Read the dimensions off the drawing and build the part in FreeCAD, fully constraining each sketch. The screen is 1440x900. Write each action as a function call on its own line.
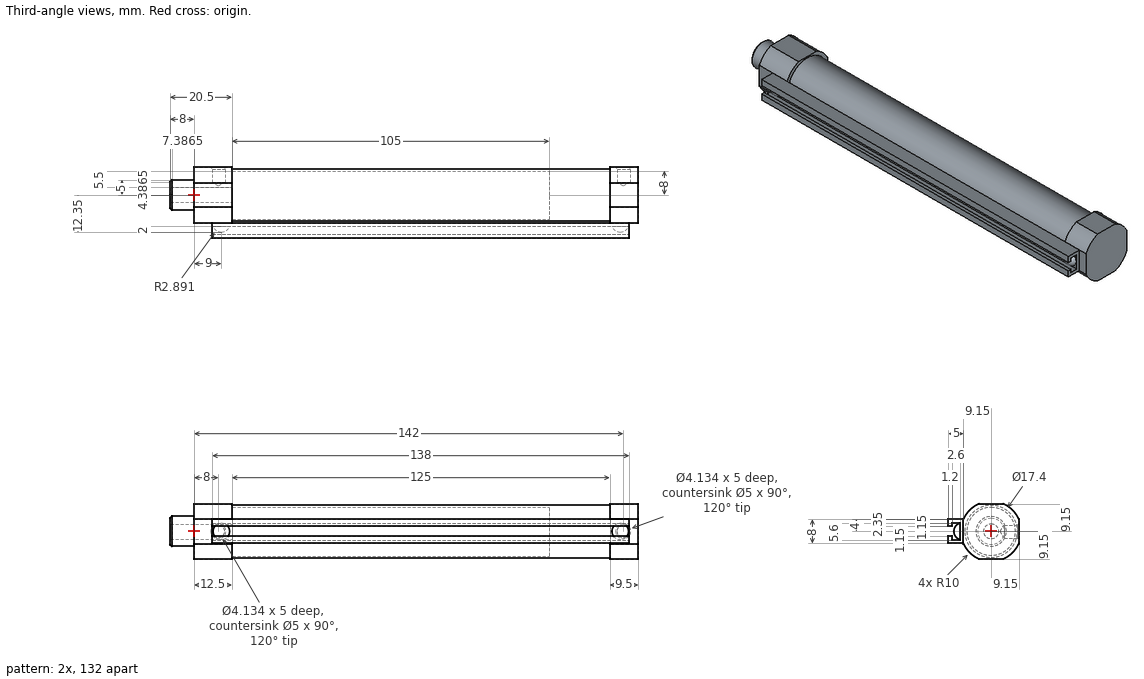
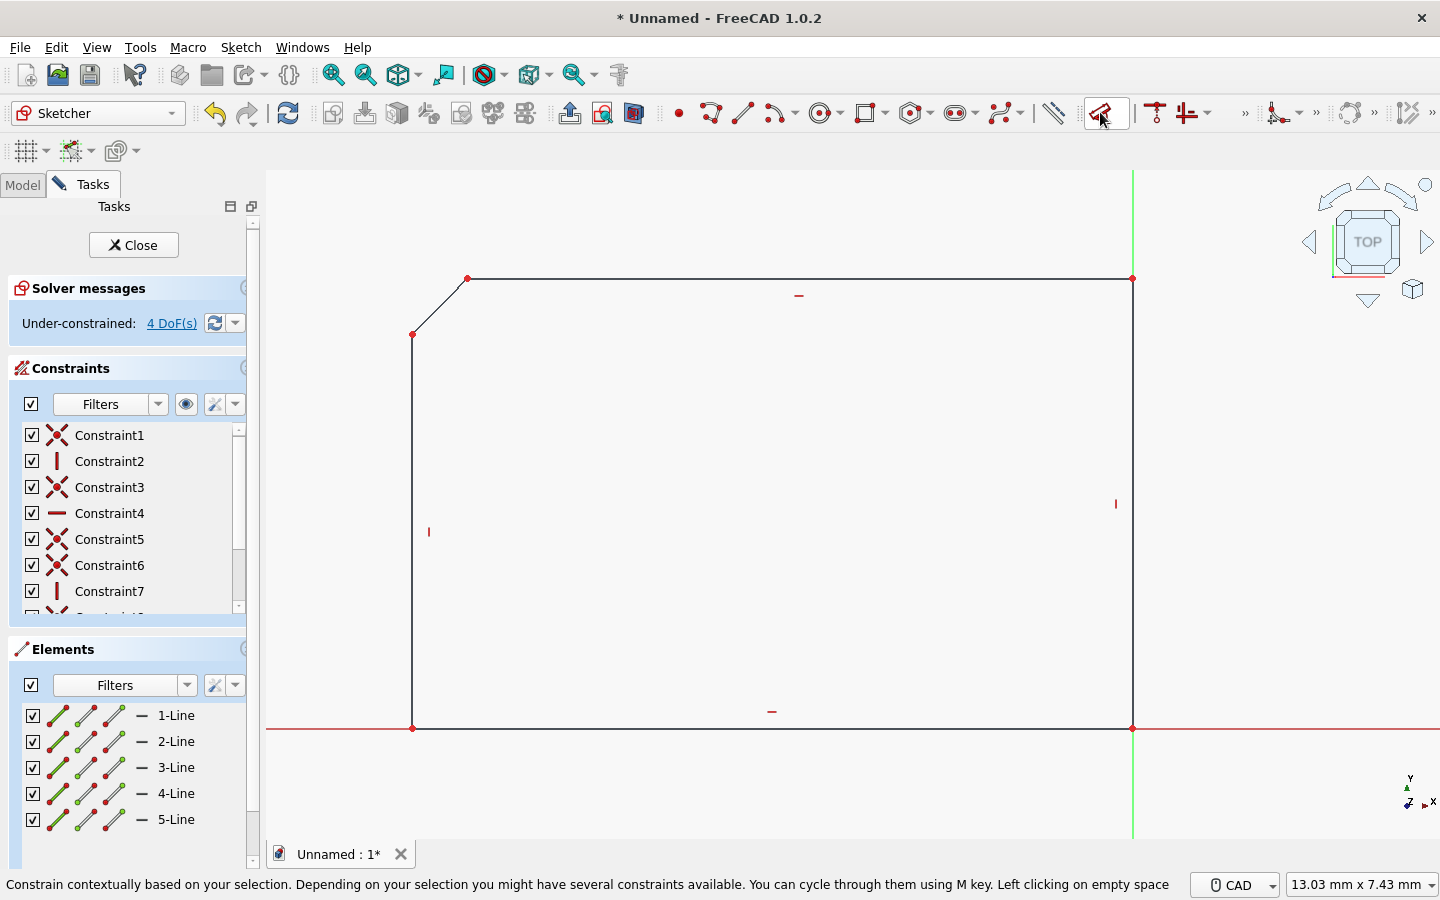
click(1133, 594)
click(1167, 504)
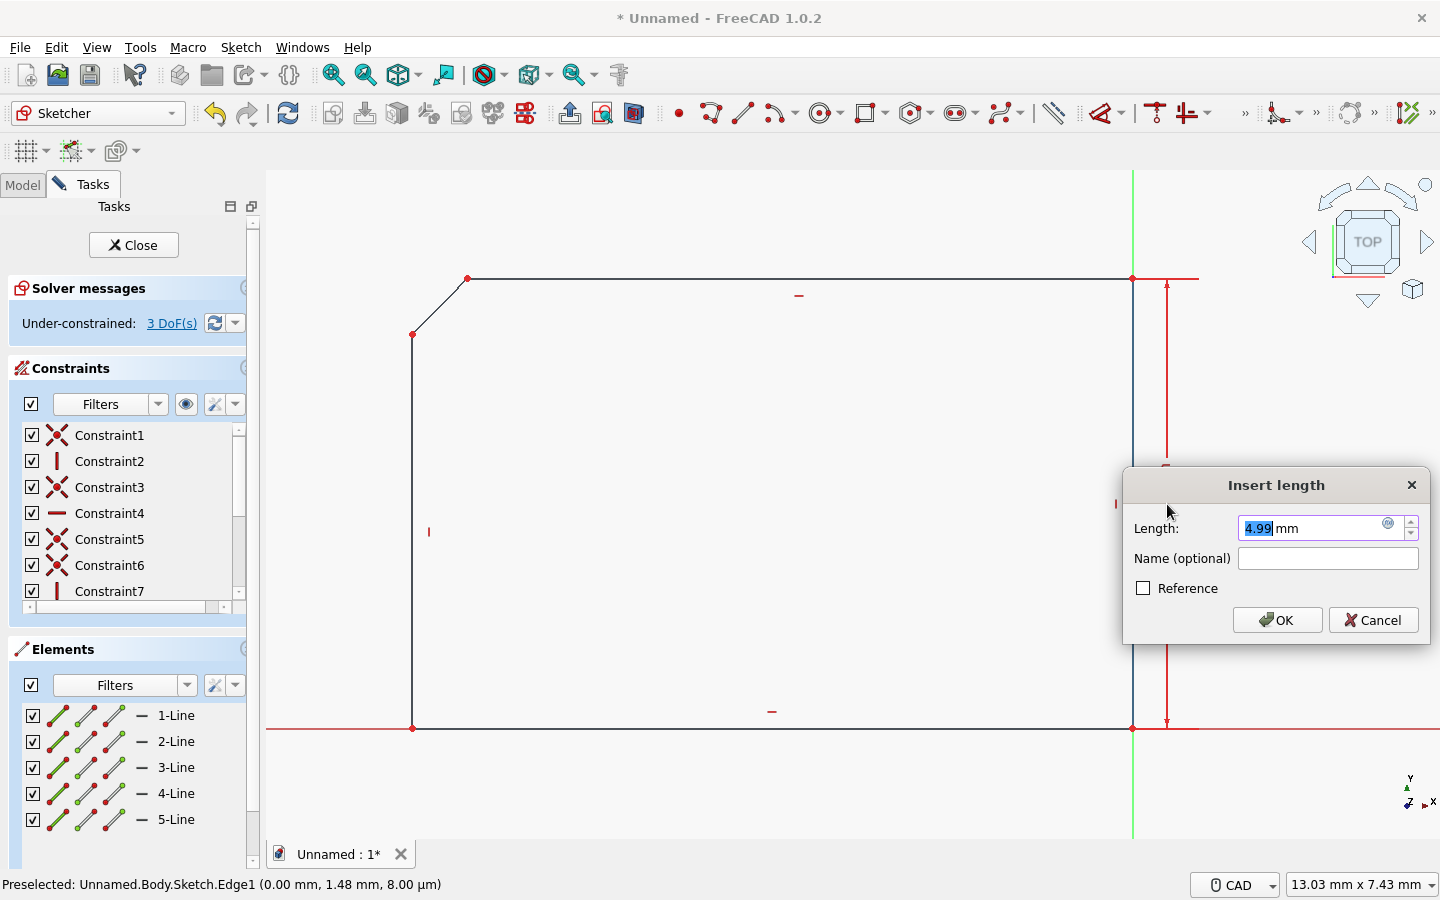
text(5)
key(Return)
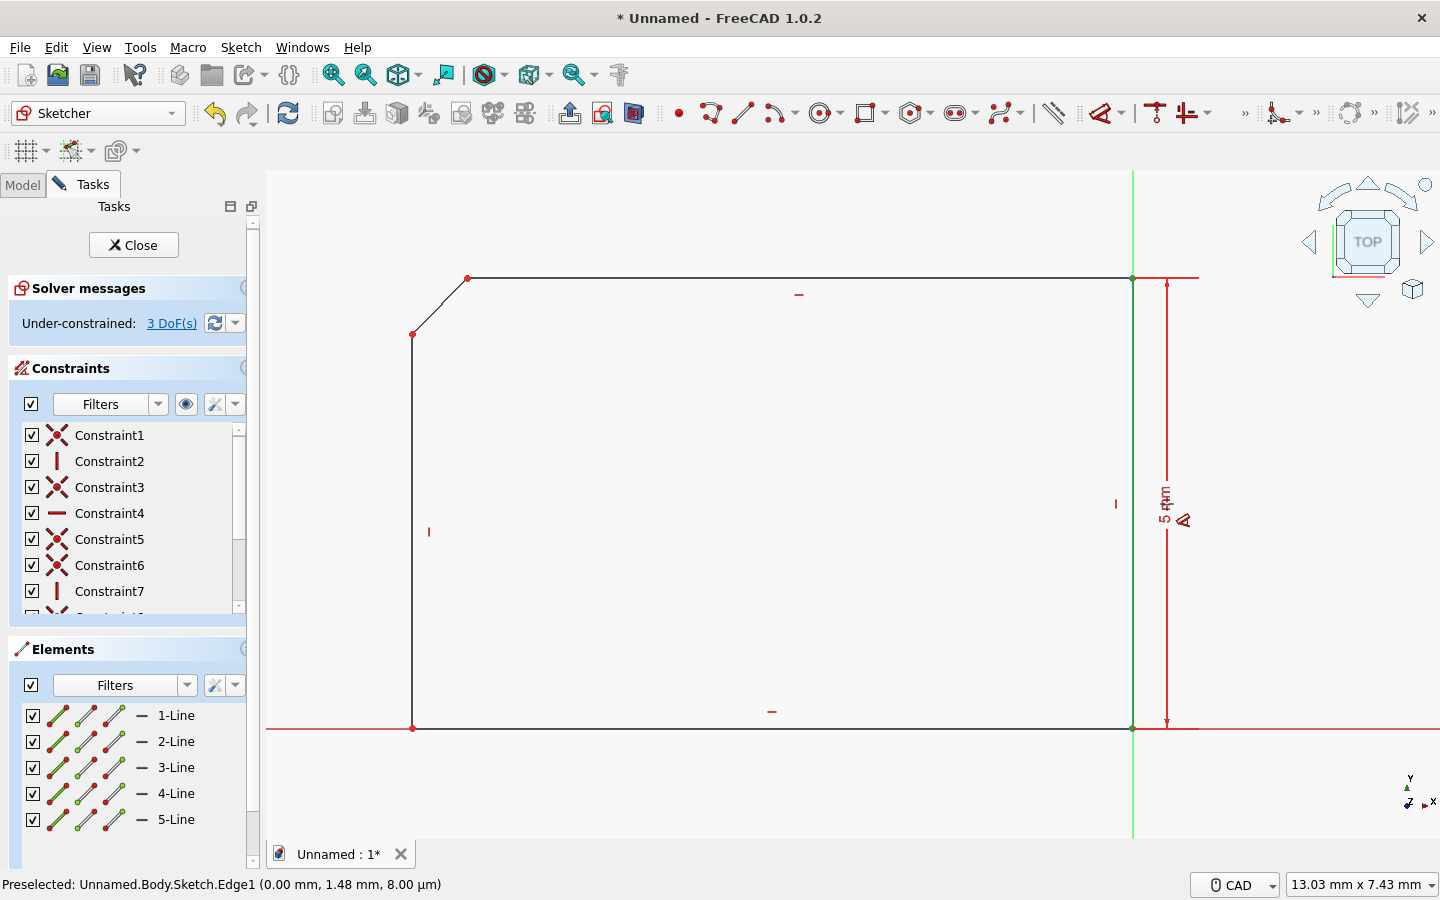
click(628, 729)
click(773, 763)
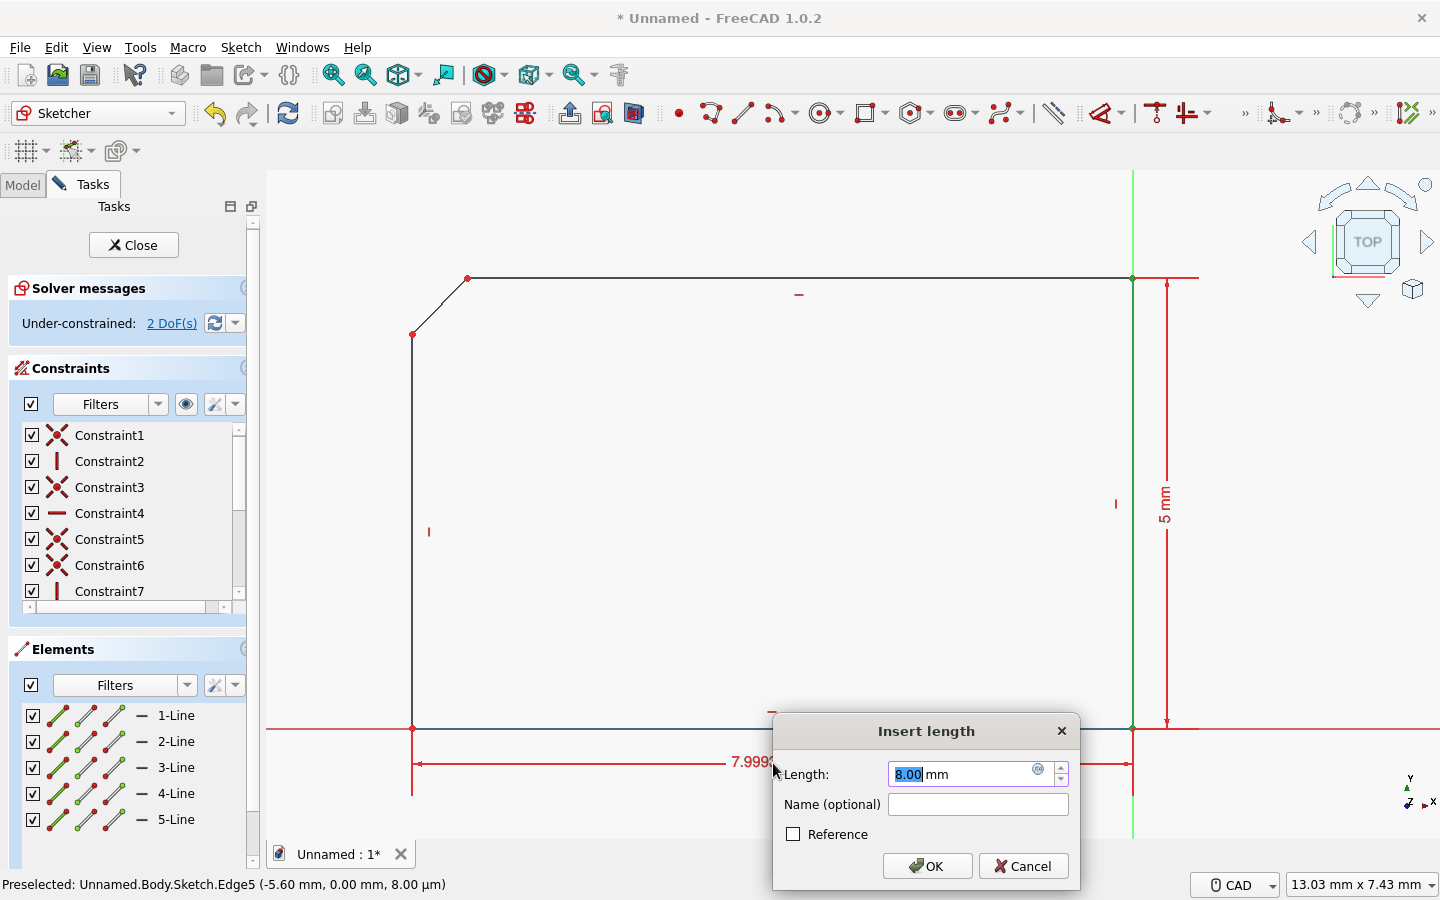
text(8)
key(Return)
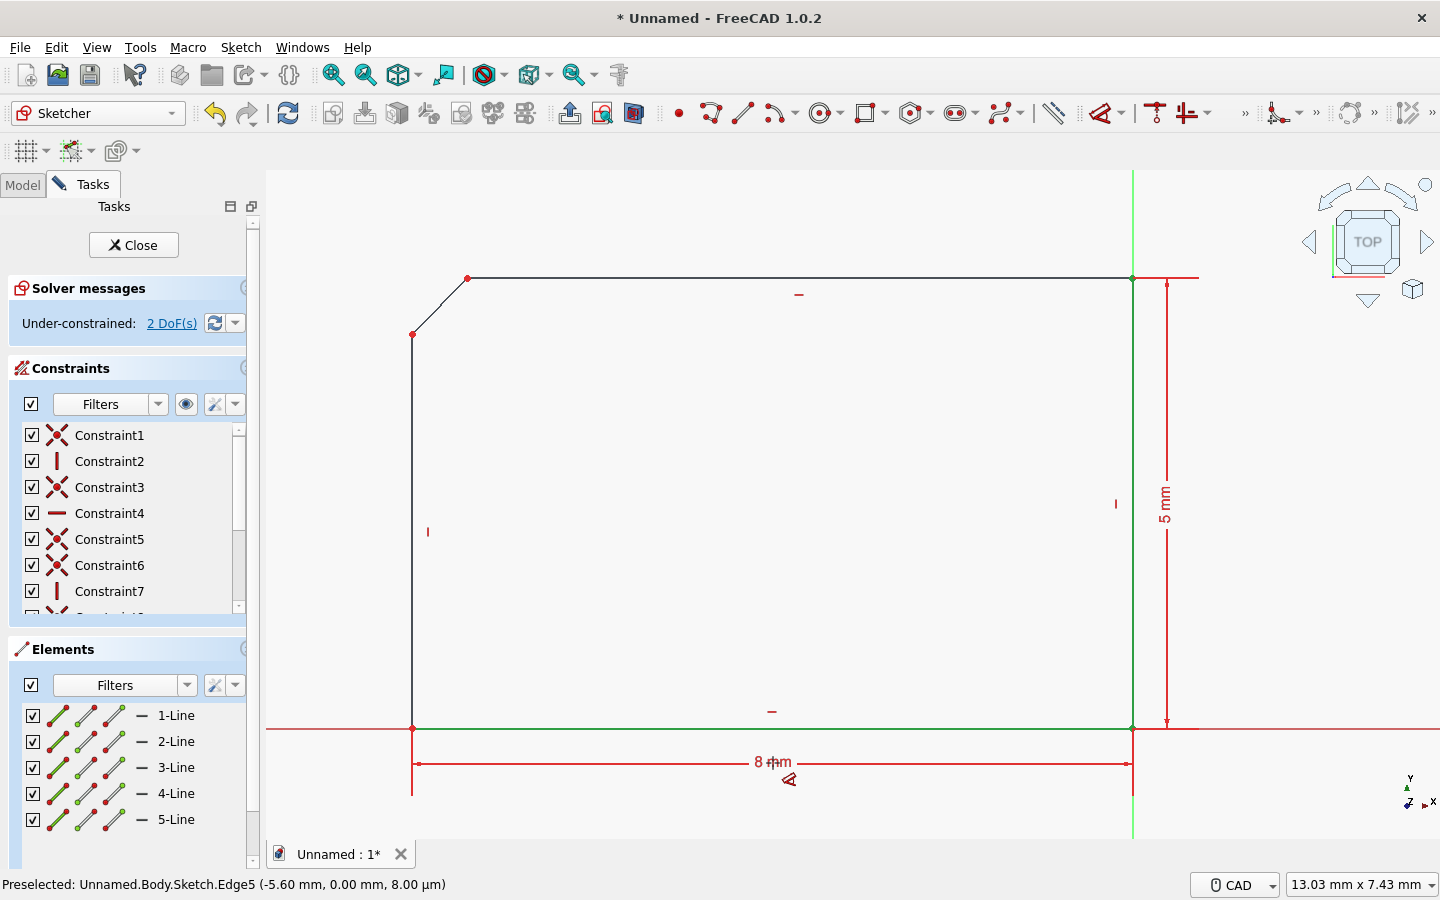
click(933, 278)
click(800, 244)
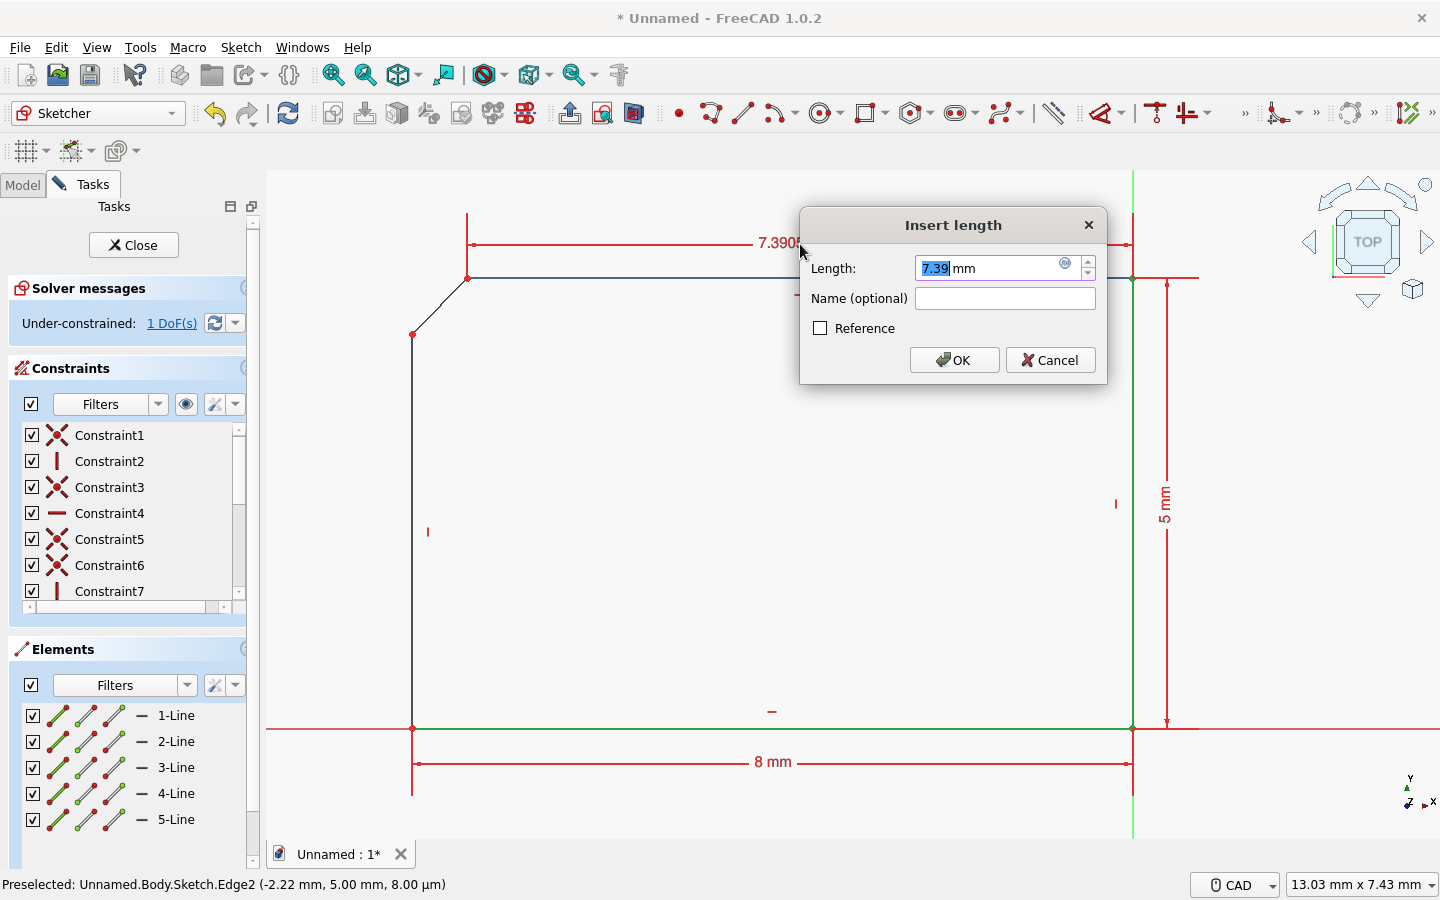
text(7.3865)
key(Return)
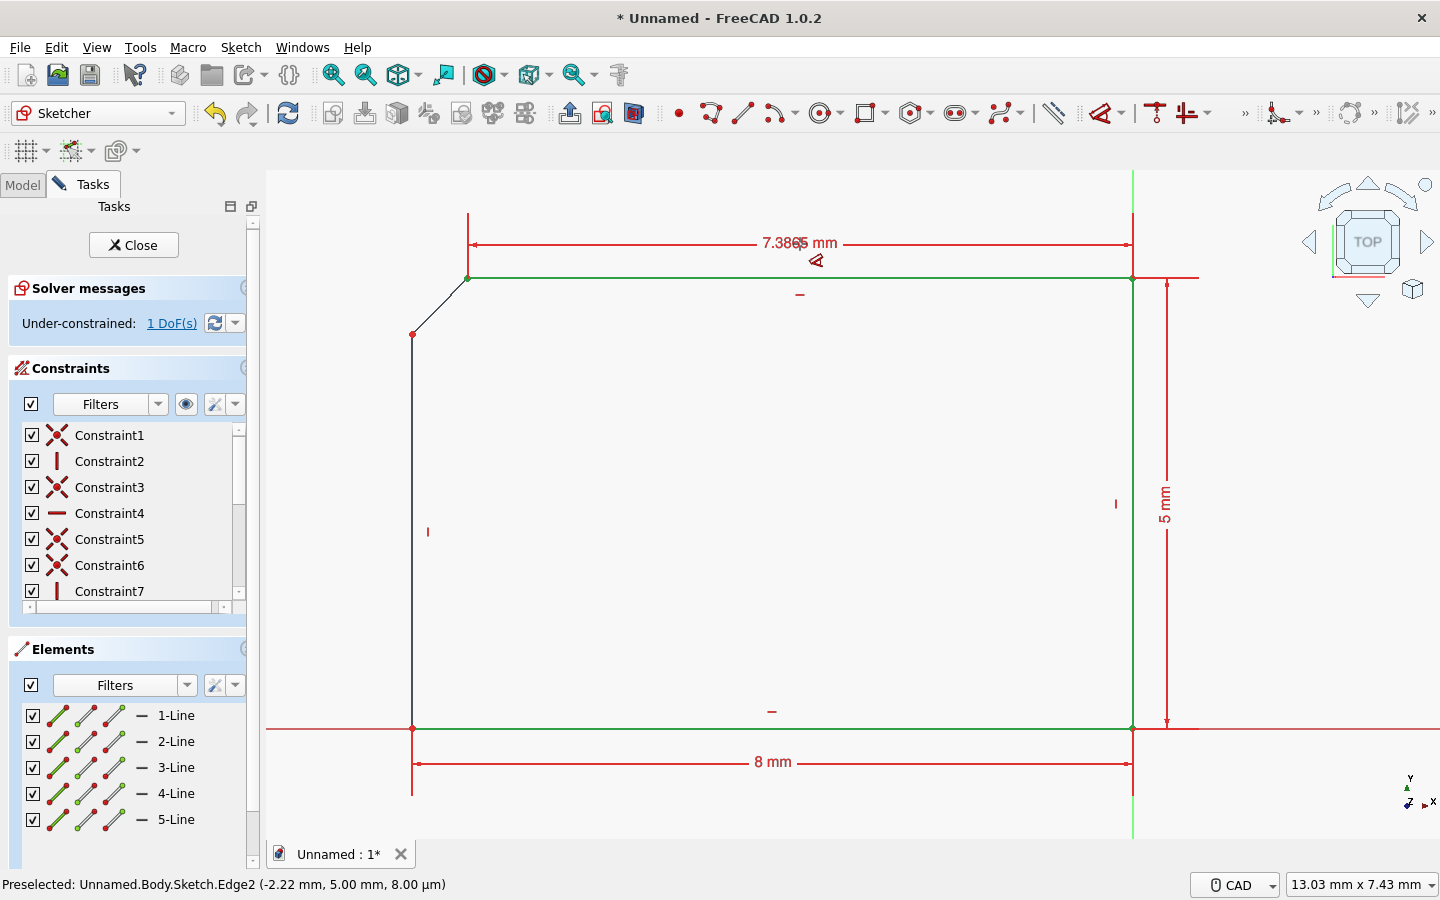
click(412, 453)
click(378, 532)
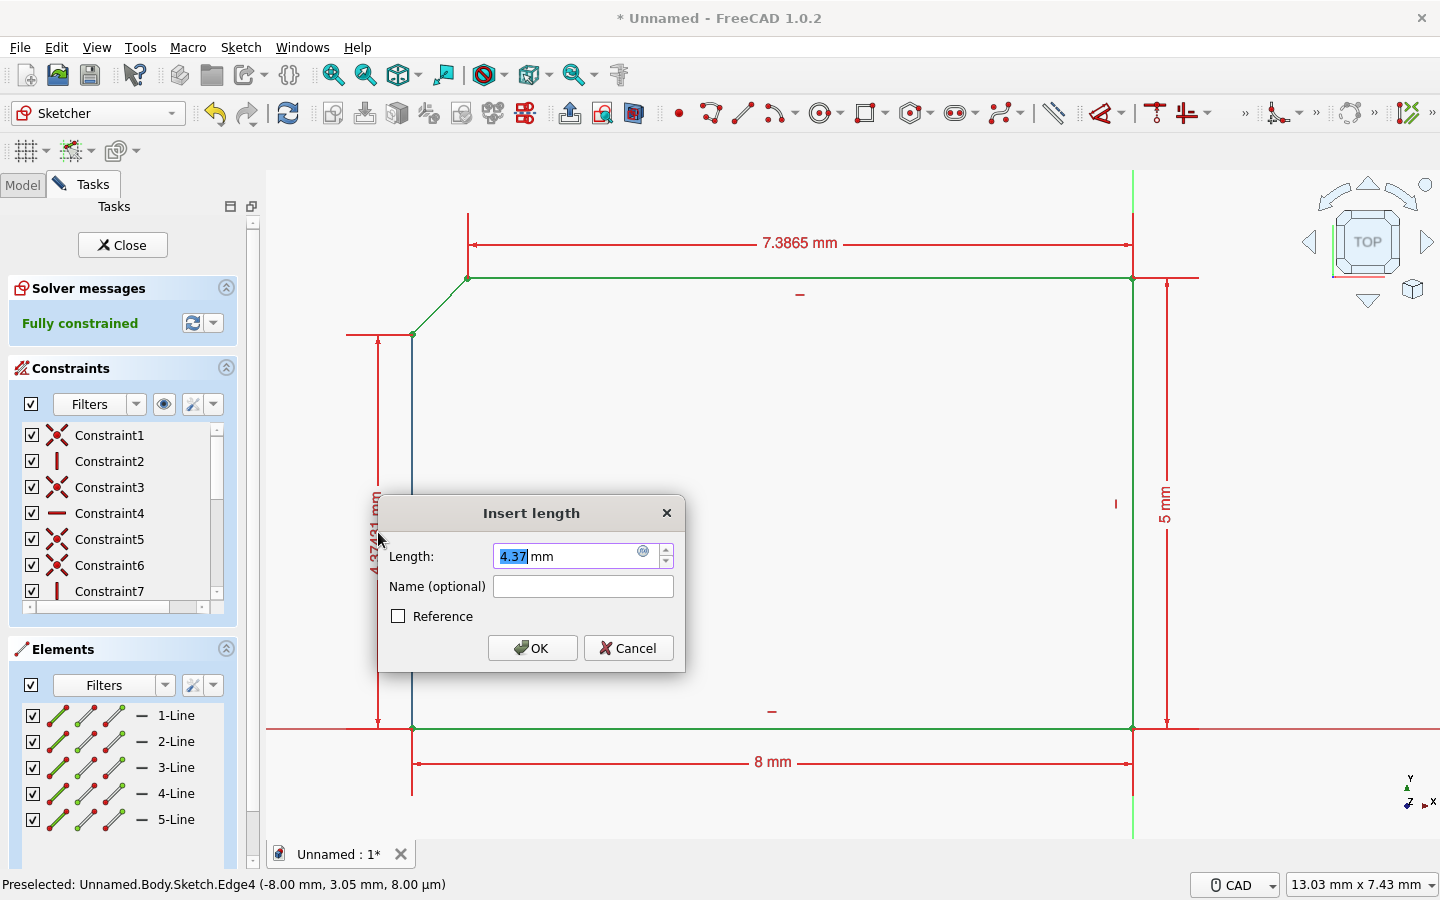
text(4.3865)
key(Return)
key(Escape)